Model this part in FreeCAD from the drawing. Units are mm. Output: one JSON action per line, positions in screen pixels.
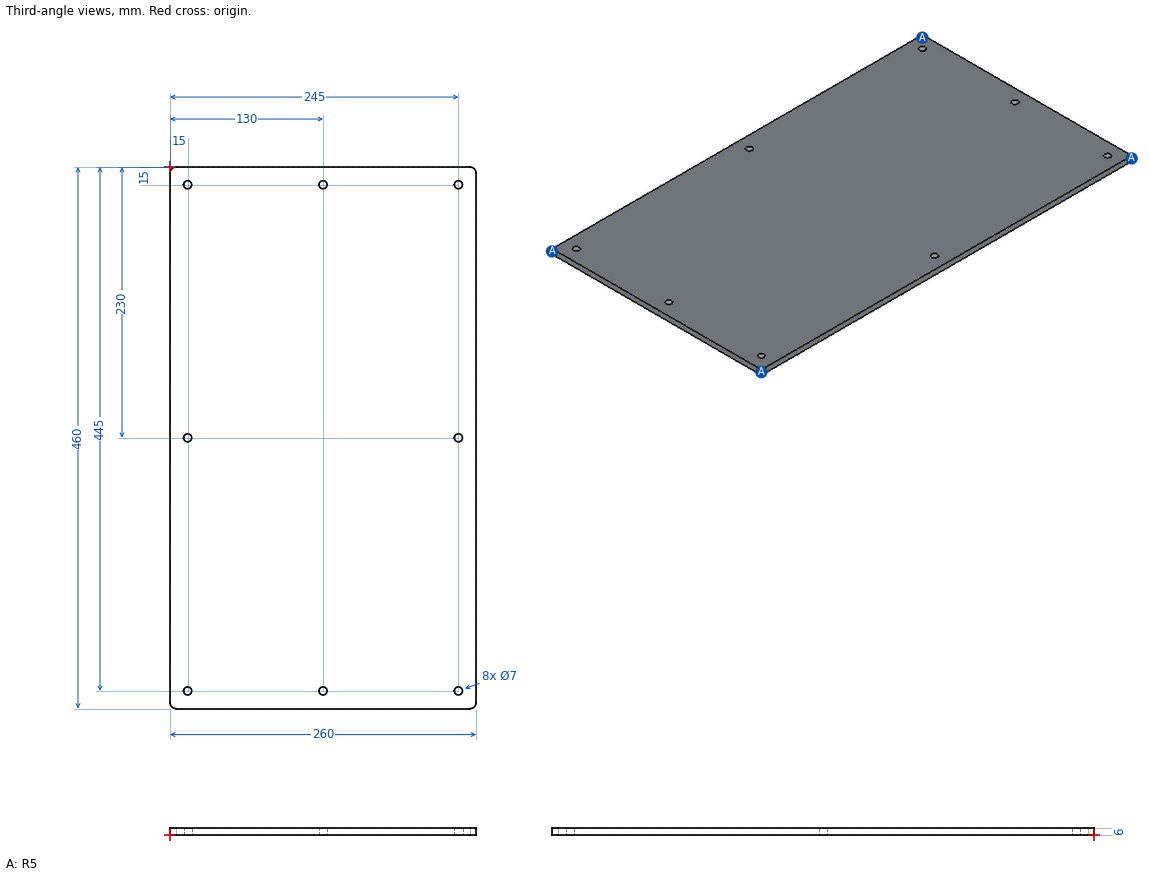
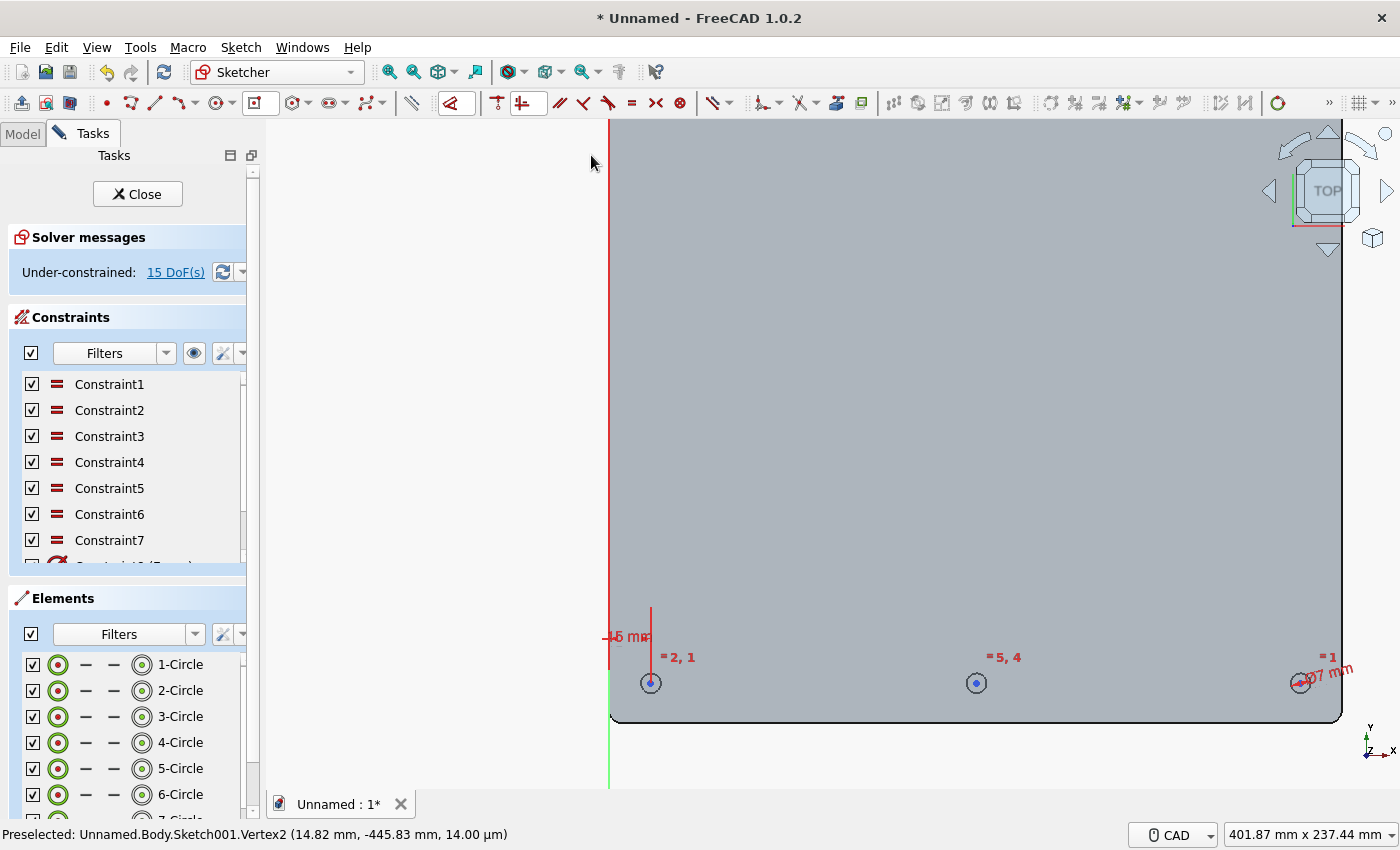
{"action": "scroll", "coordinate": [651, 684], "scroll_direction": "down", "scroll_amount": 5}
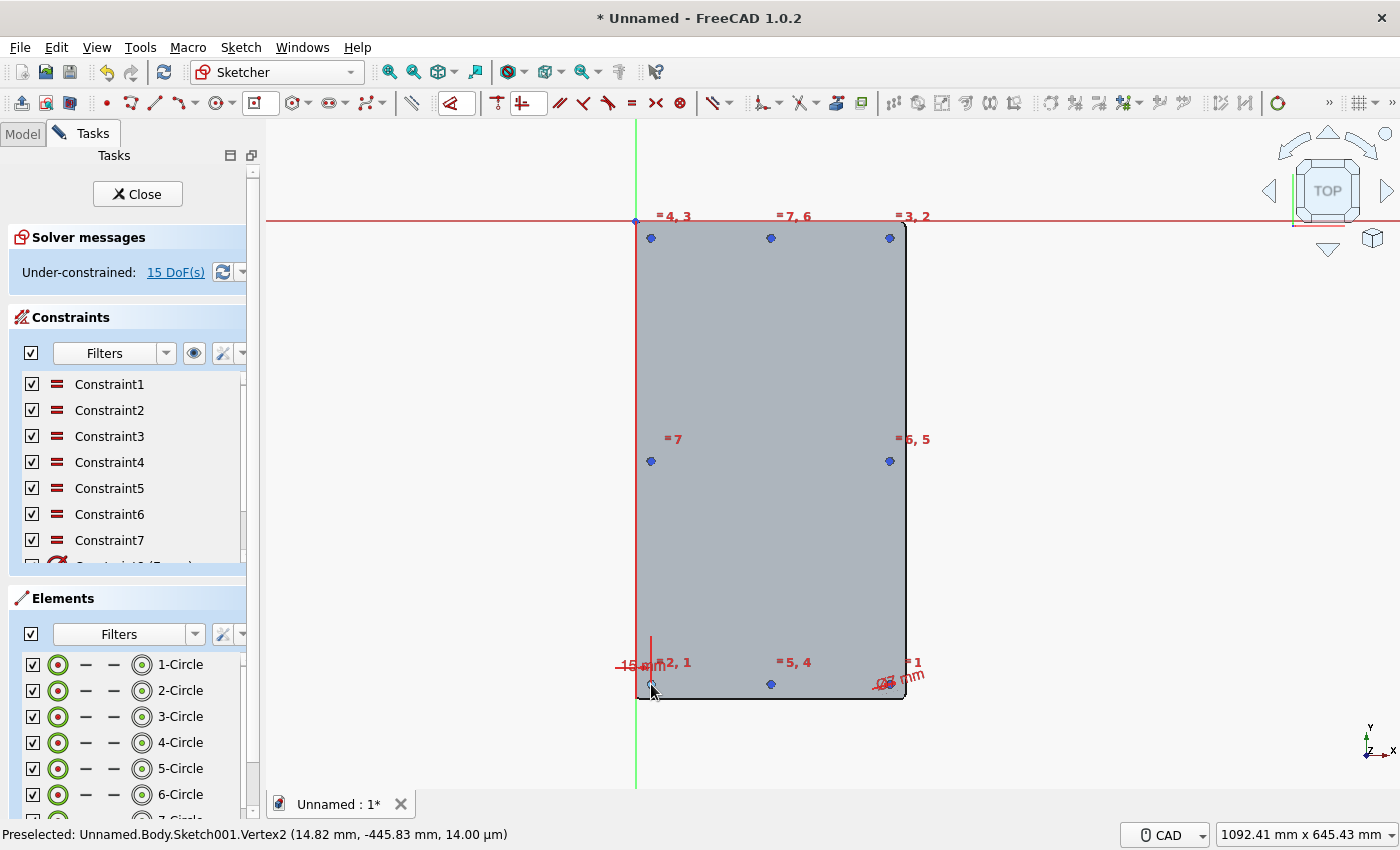
{"action": "scroll", "coordinate": [890, 238], "scroll_direction": "up", "scroll_amount": 5}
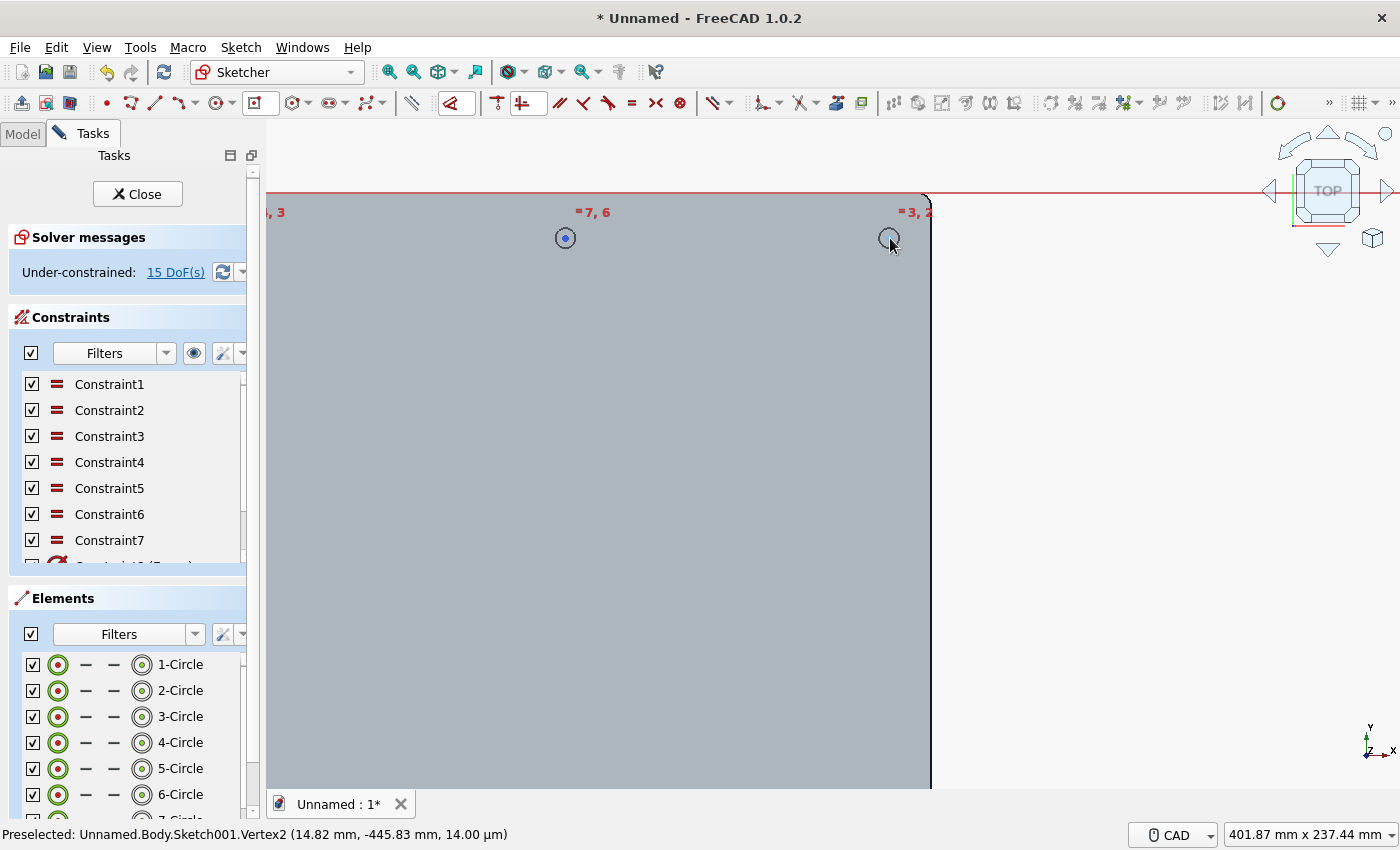
{"action": "left_click", "coordinate": [889, 238]}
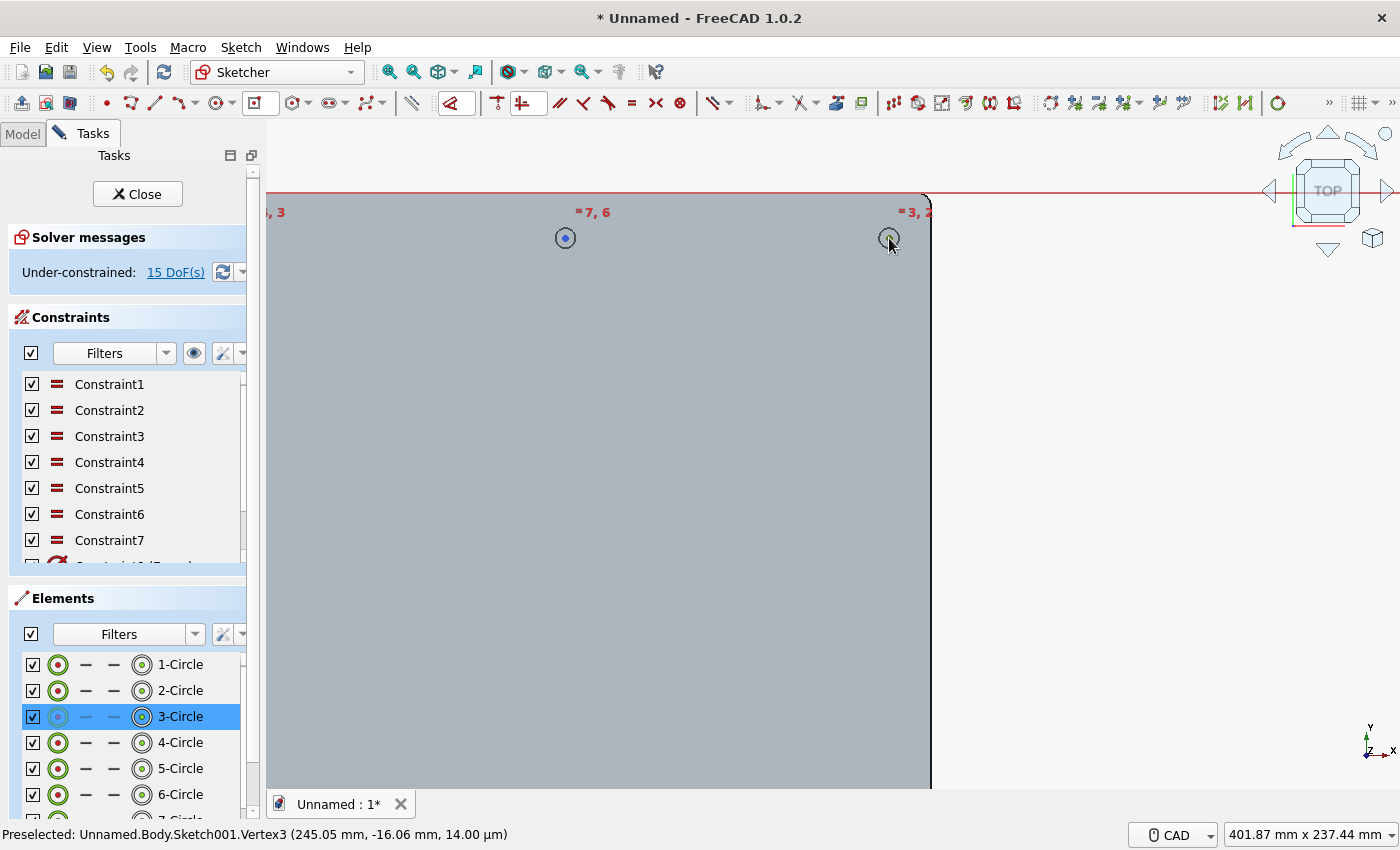
{"action": "key", "text": "i"}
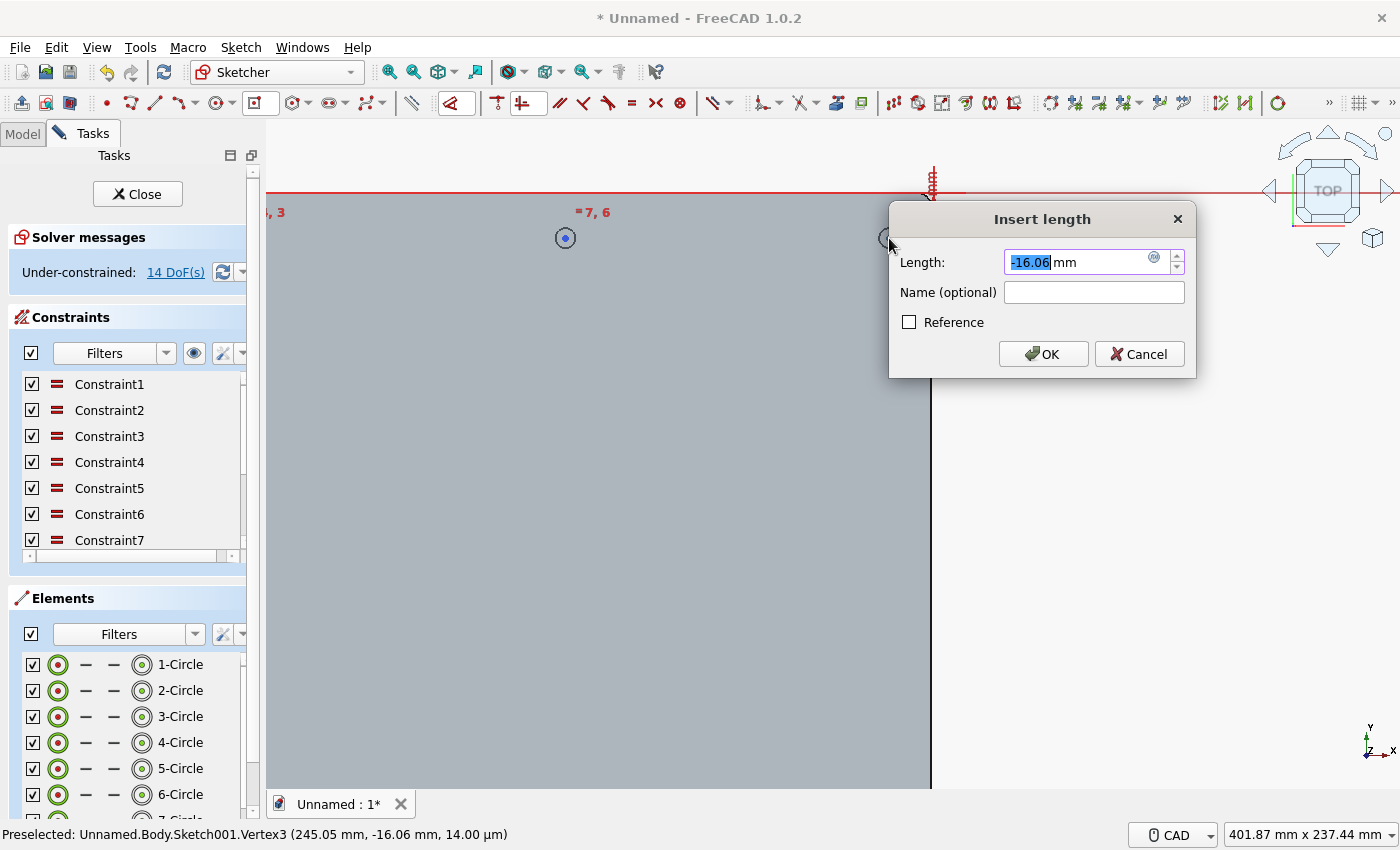
{"action": "type", "text": "-15"}
{"action": "key", "text": "Return"}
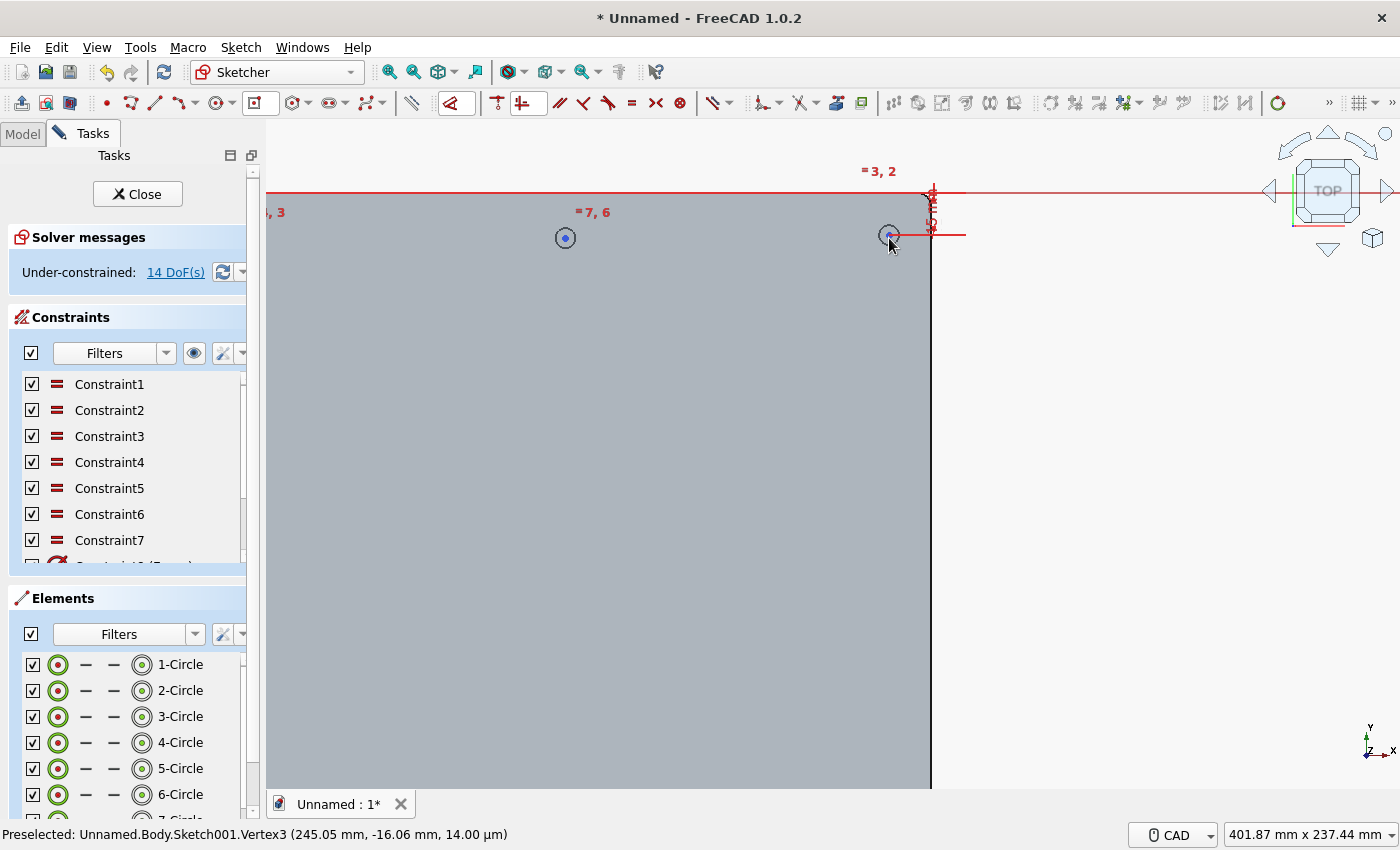
{"action": "scroll", "coordinate": [890, 238], "scroll_direction": "down", "scroll_amount": 5}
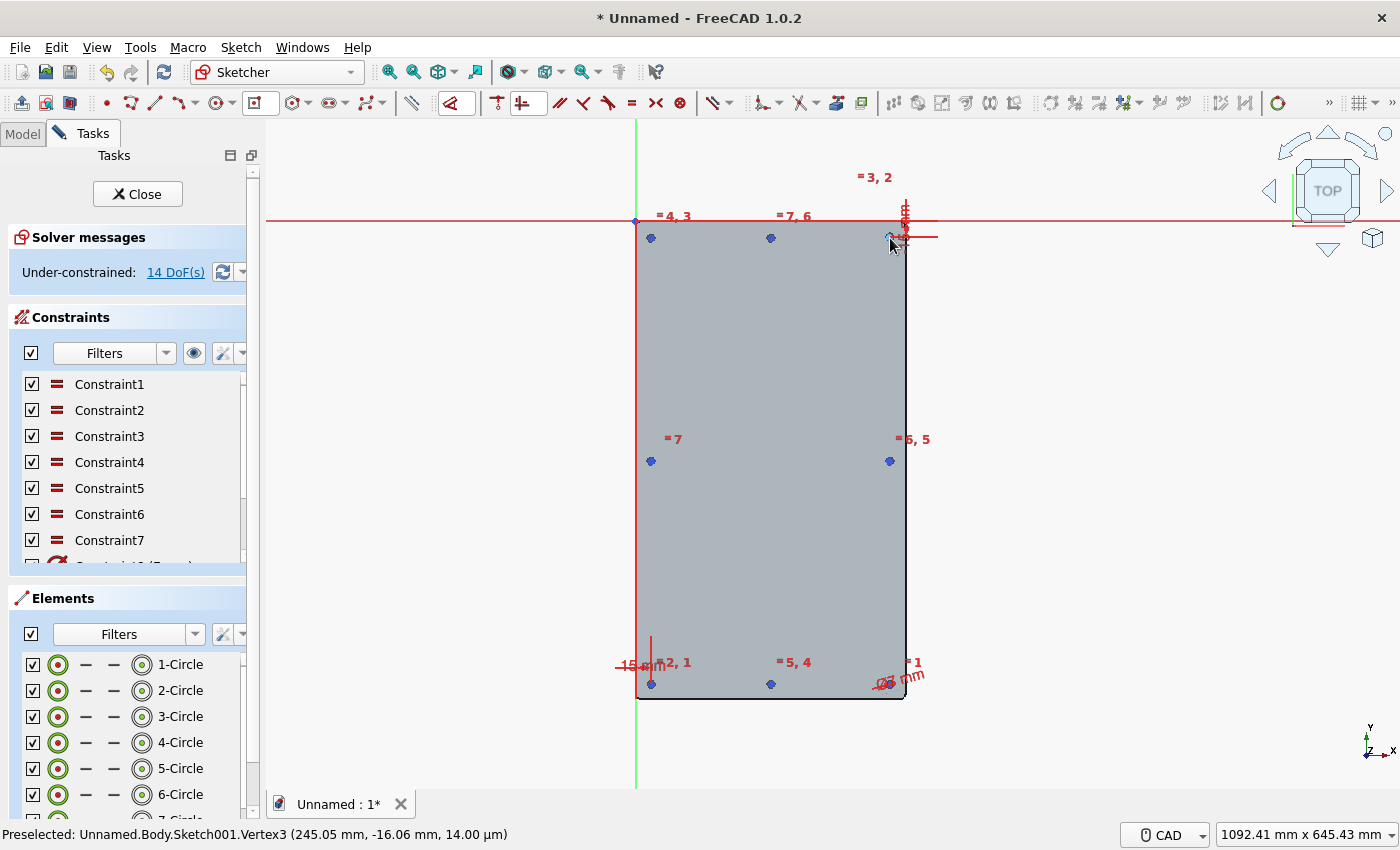
{"action": "scroll", "coordinate": [651, 238], "scroll_direction": "up", "scroll_amount": 5}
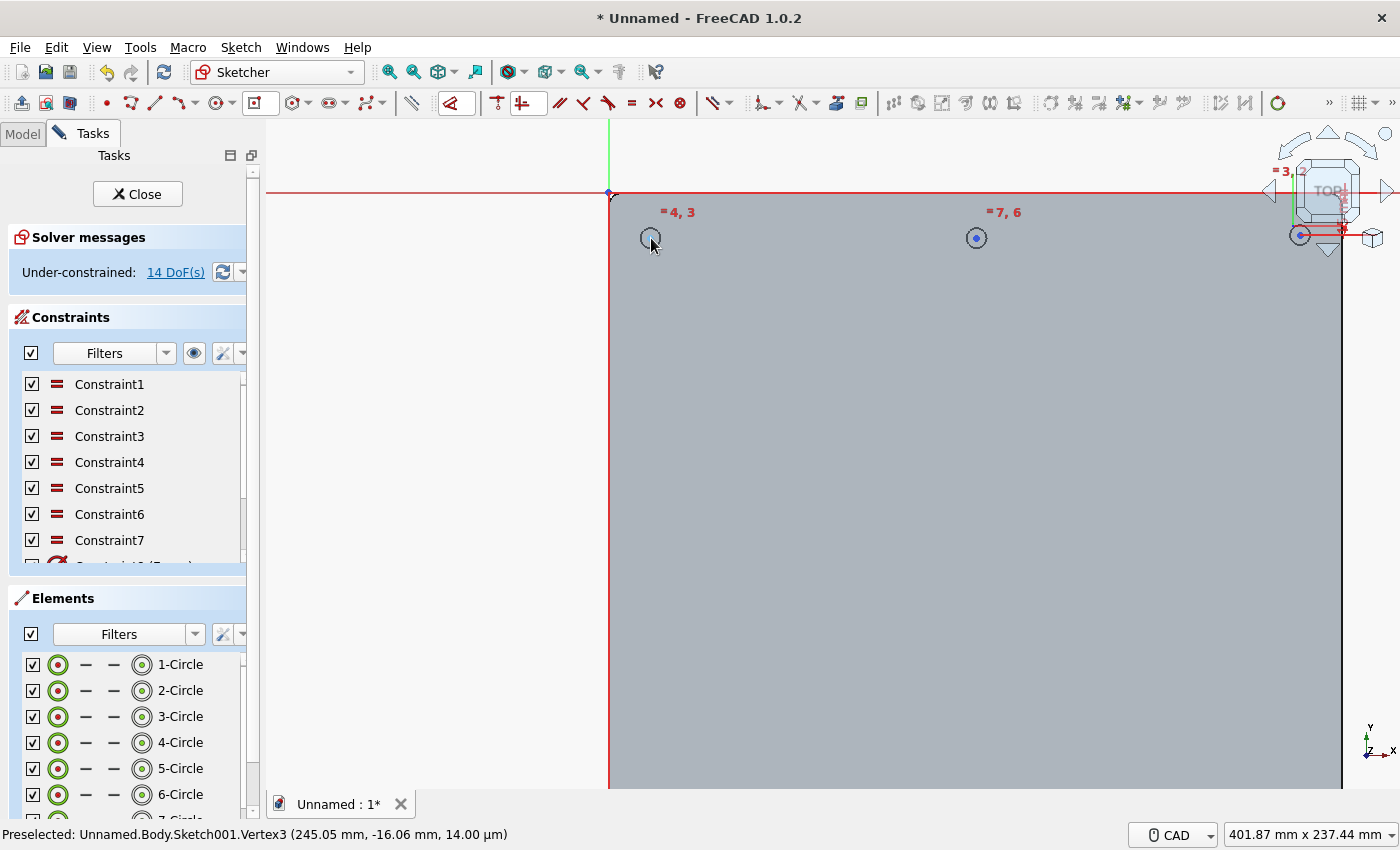
{"action": "left_click", "coordinate": [650, 238]}